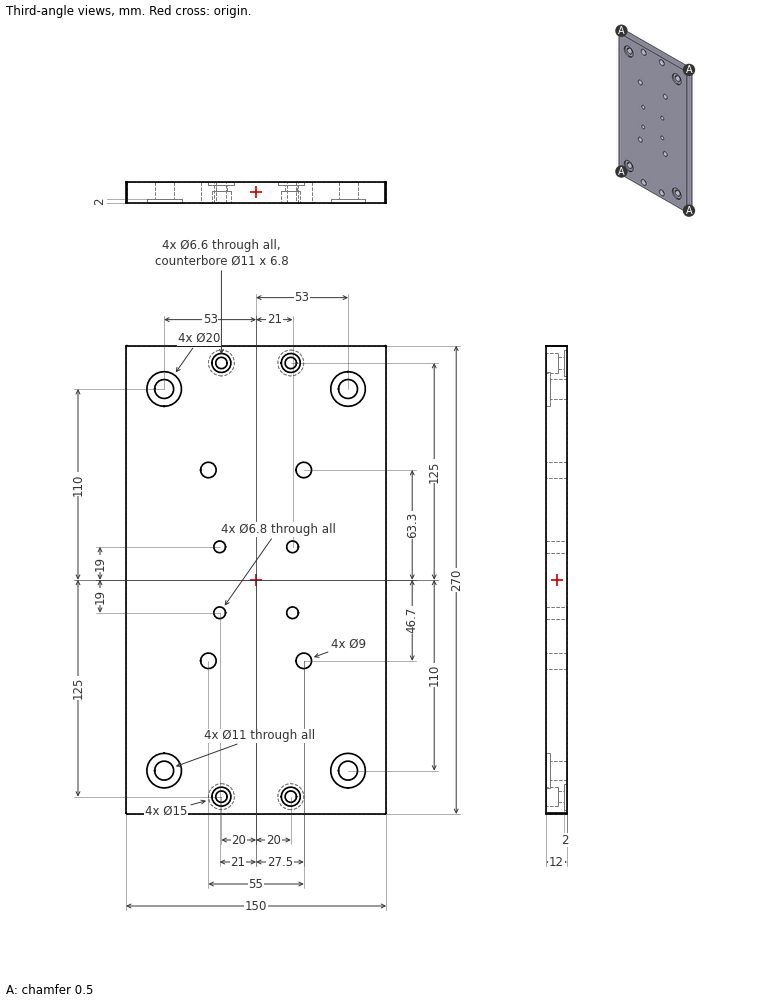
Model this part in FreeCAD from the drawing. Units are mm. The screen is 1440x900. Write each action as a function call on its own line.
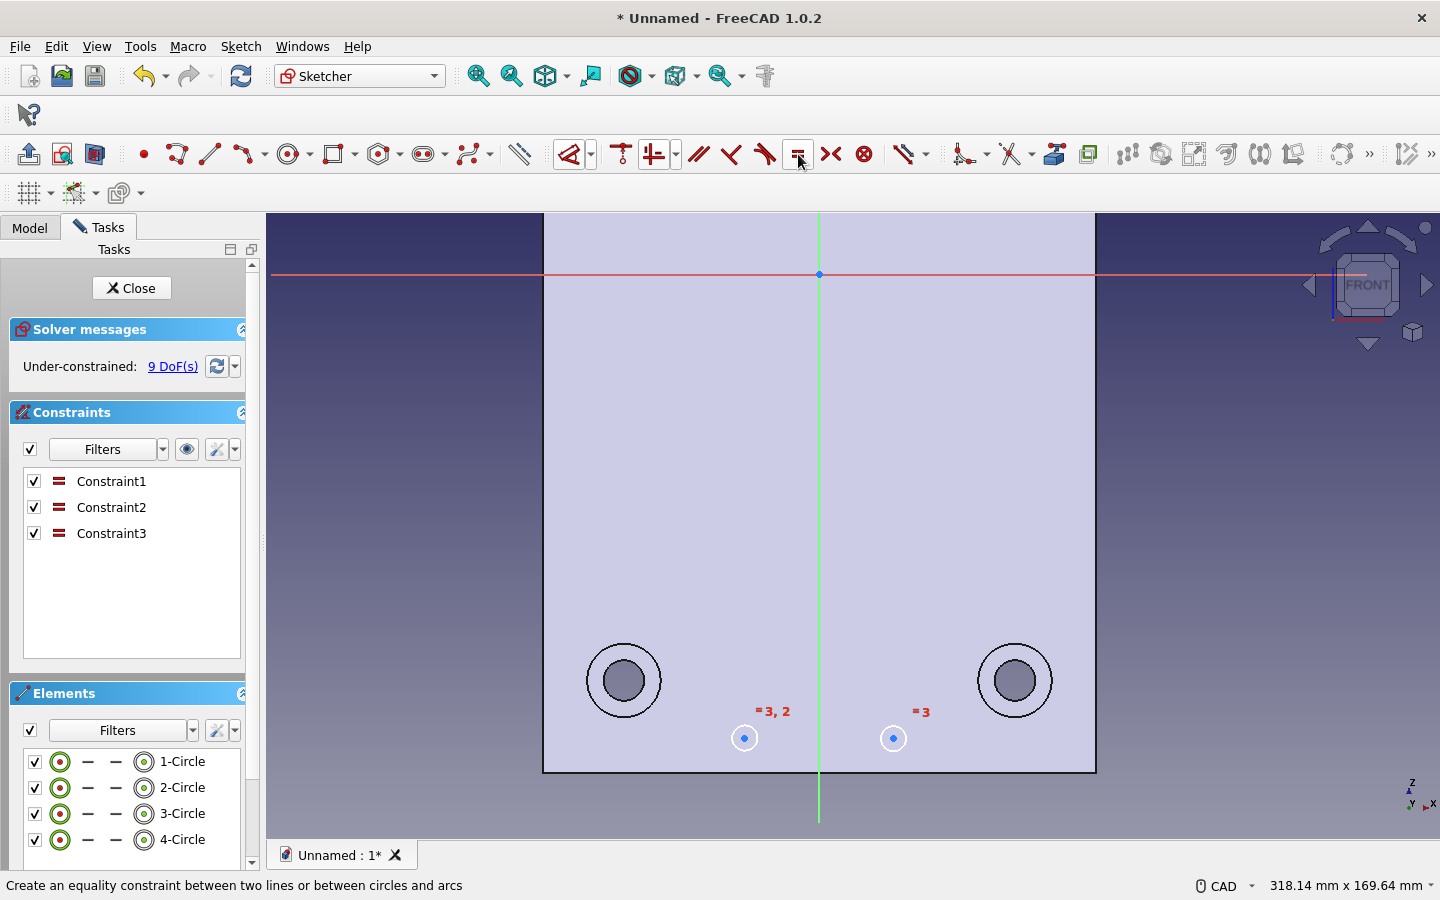
scroll(756, 731, down, 4)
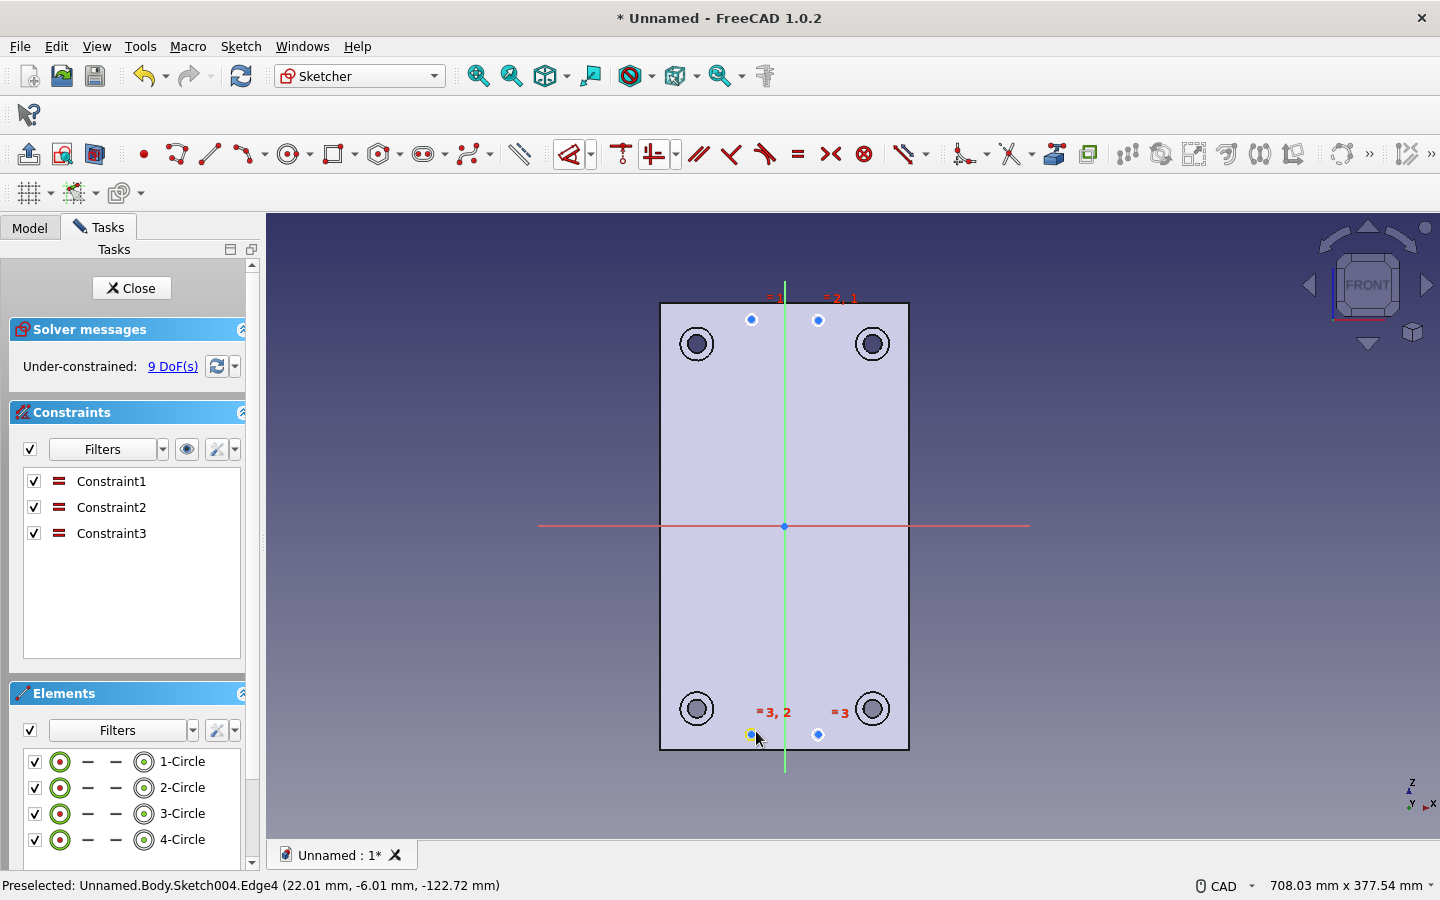
click(752, 320)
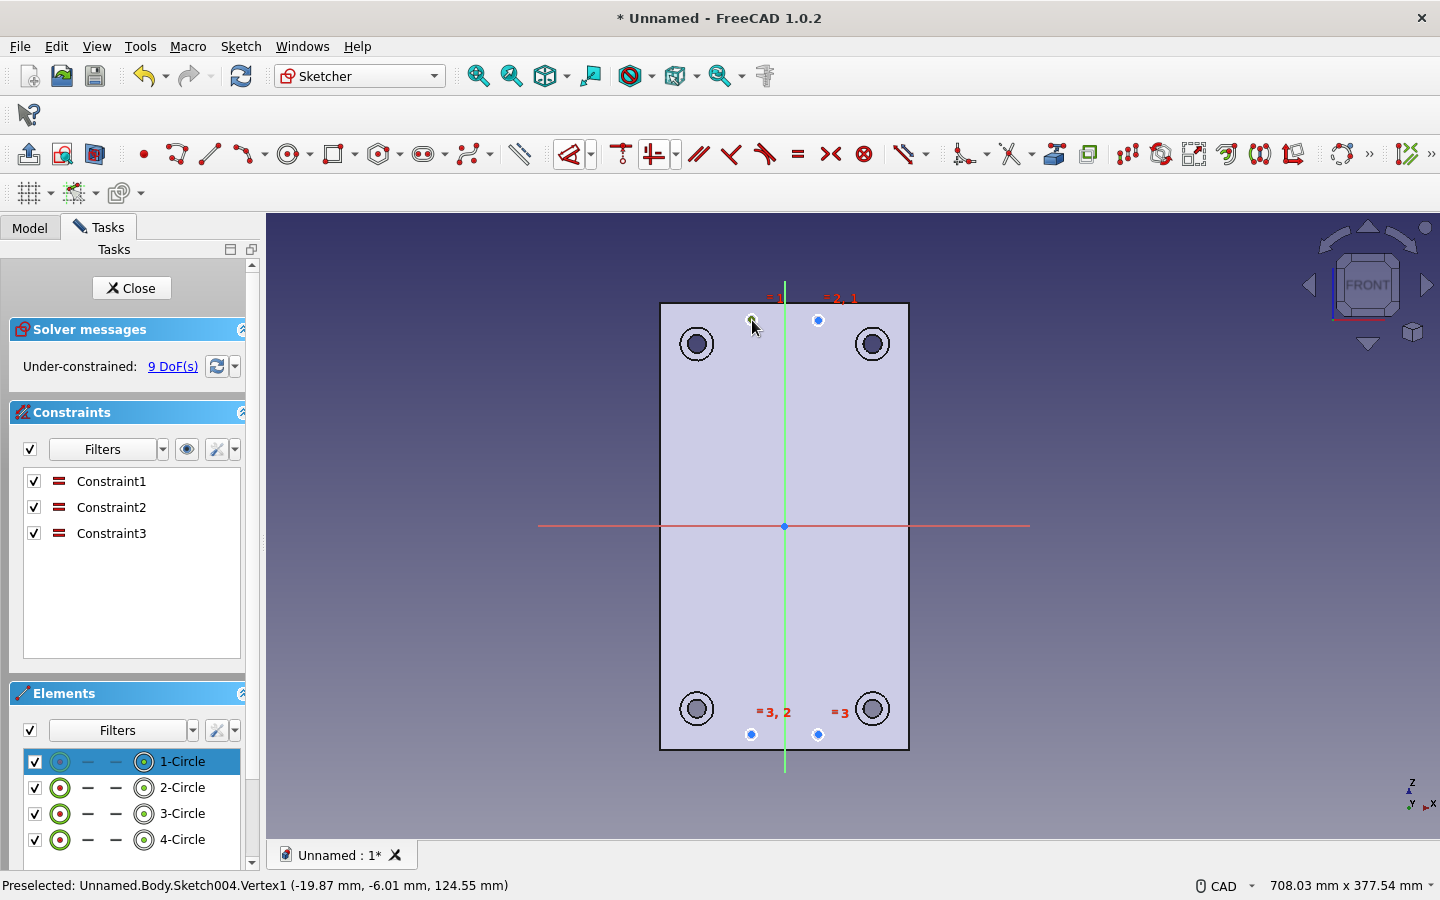
click(818, 320)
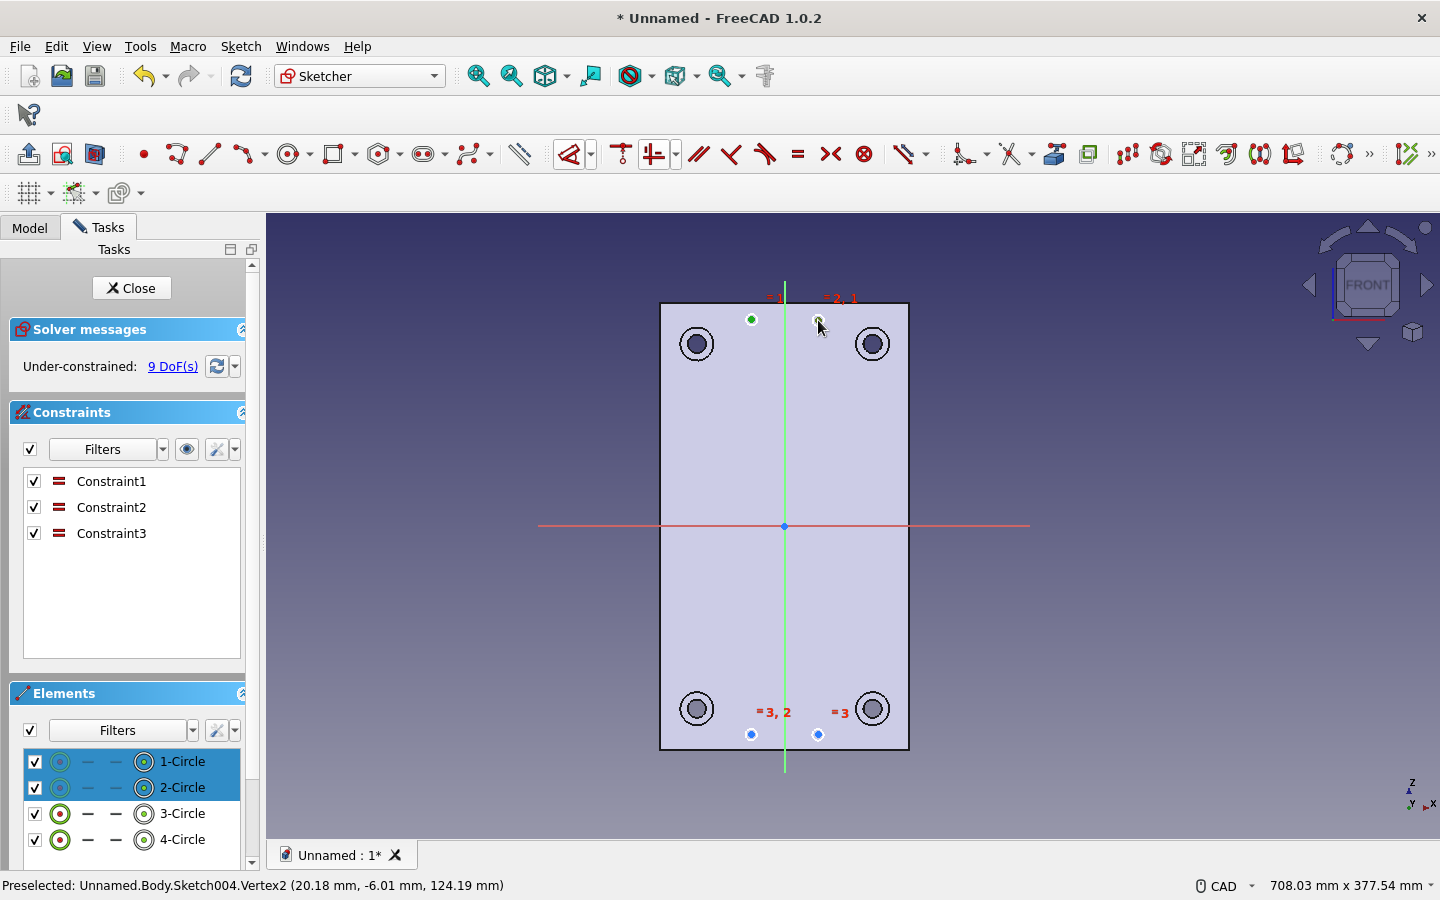
key(h)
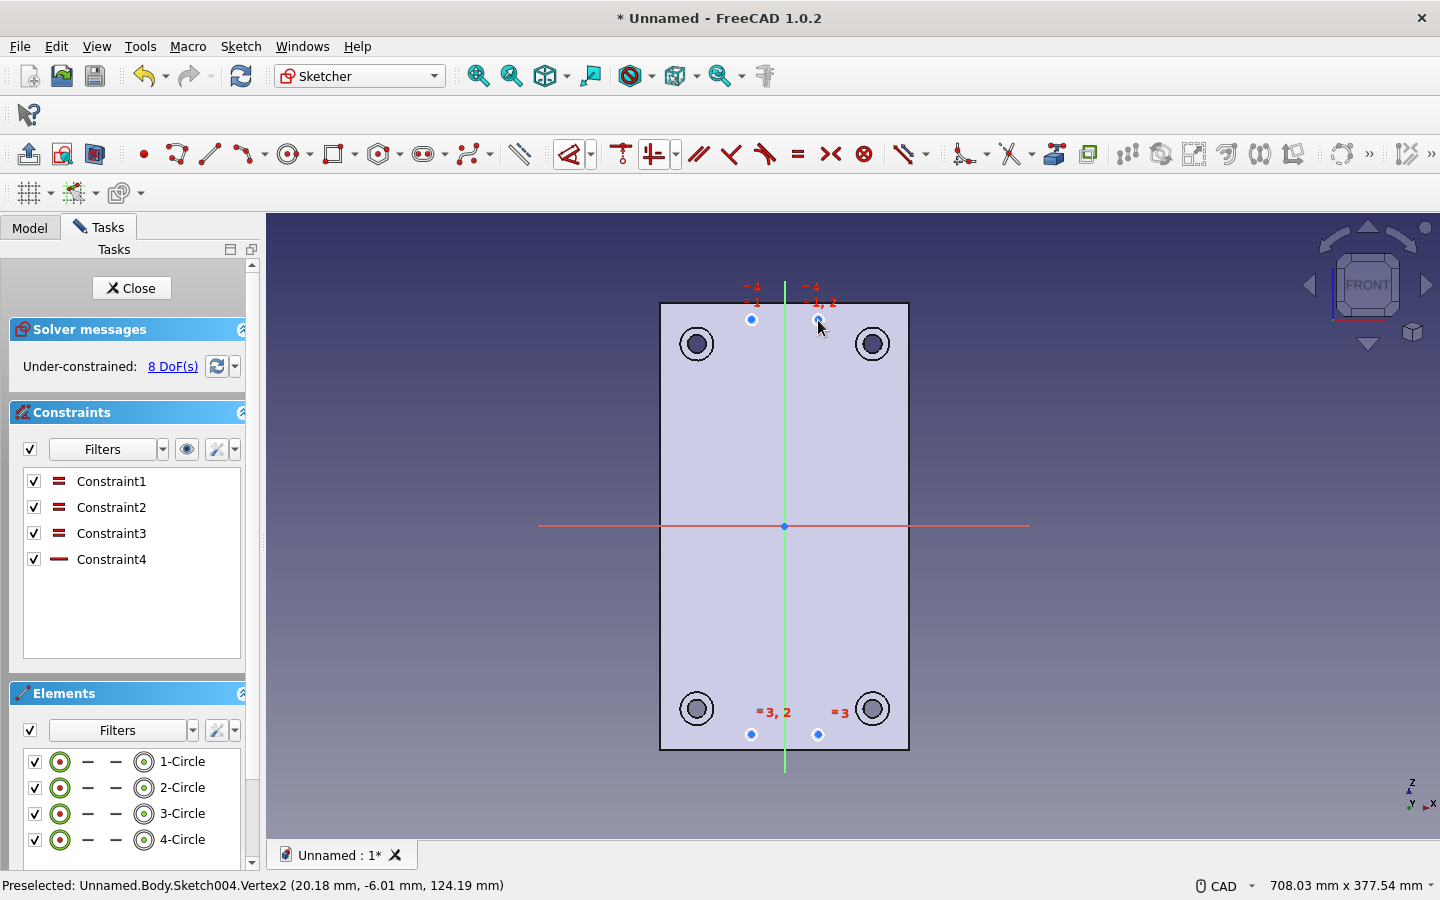
click(752, 320)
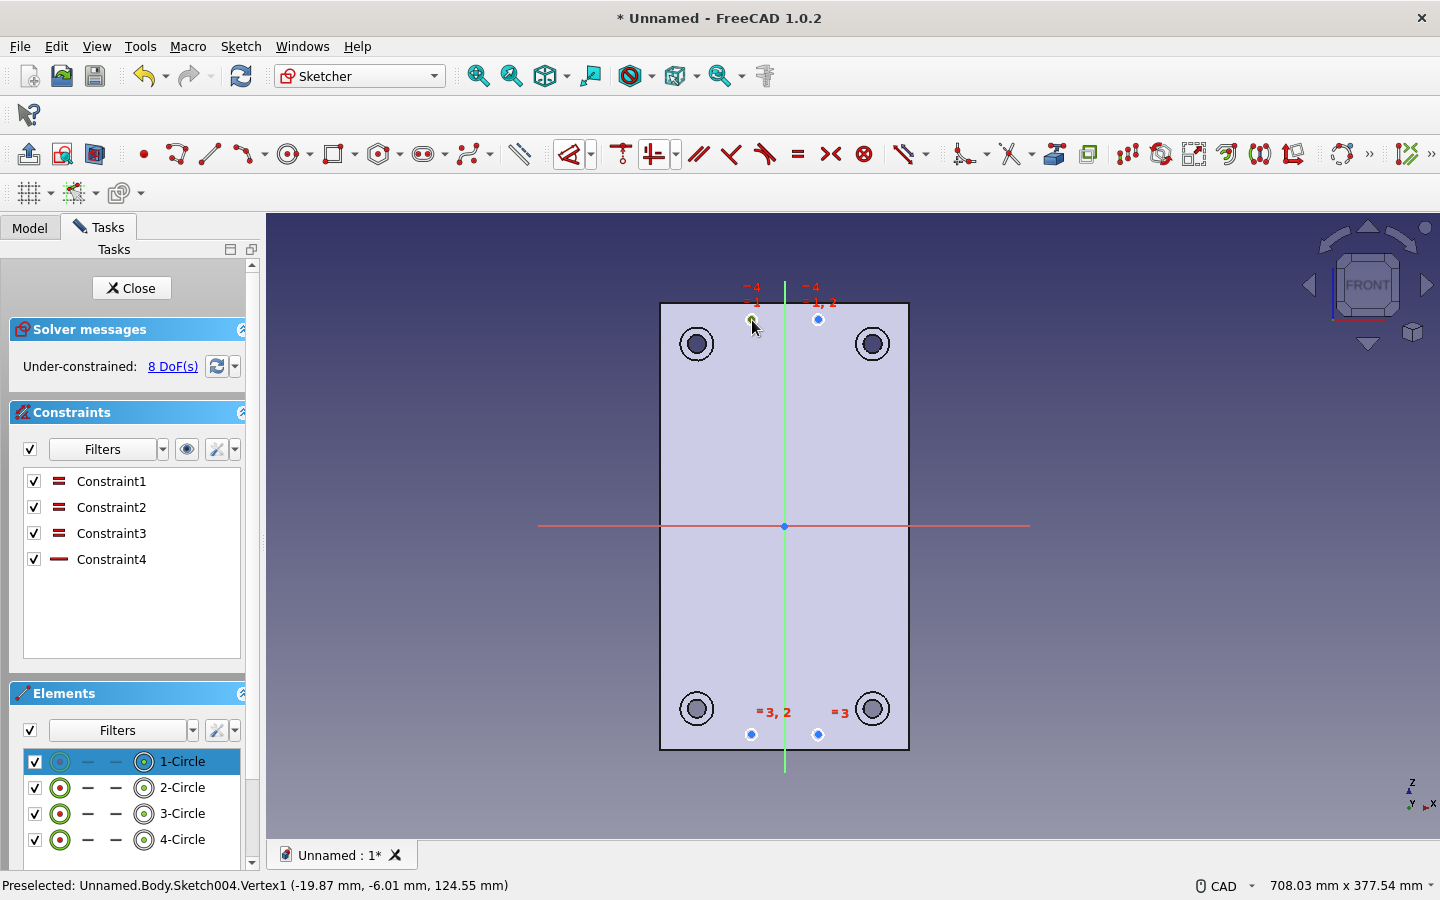
click(751, 735)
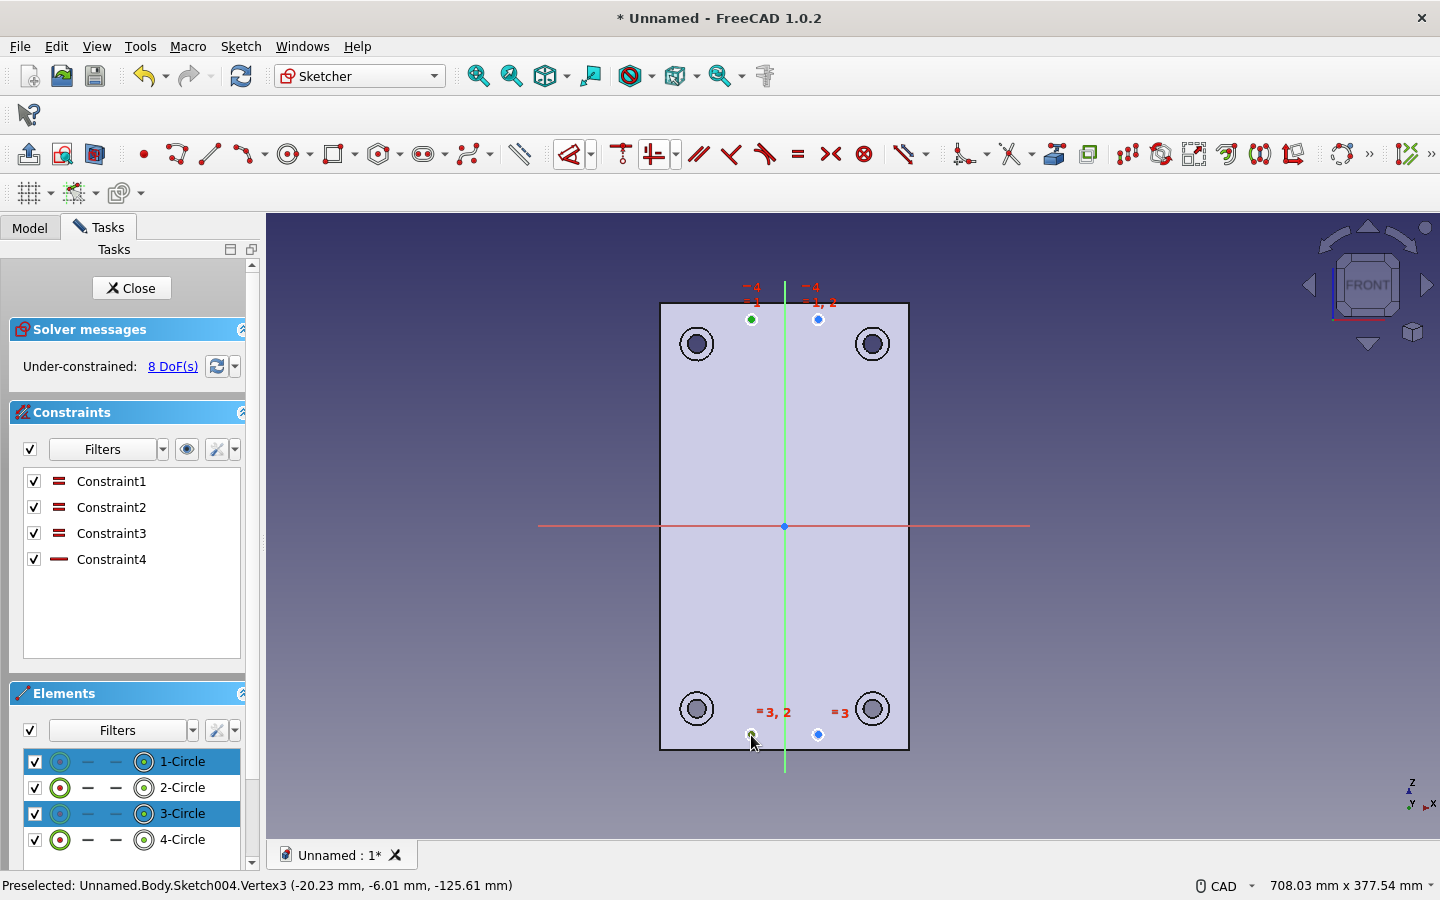
key(v)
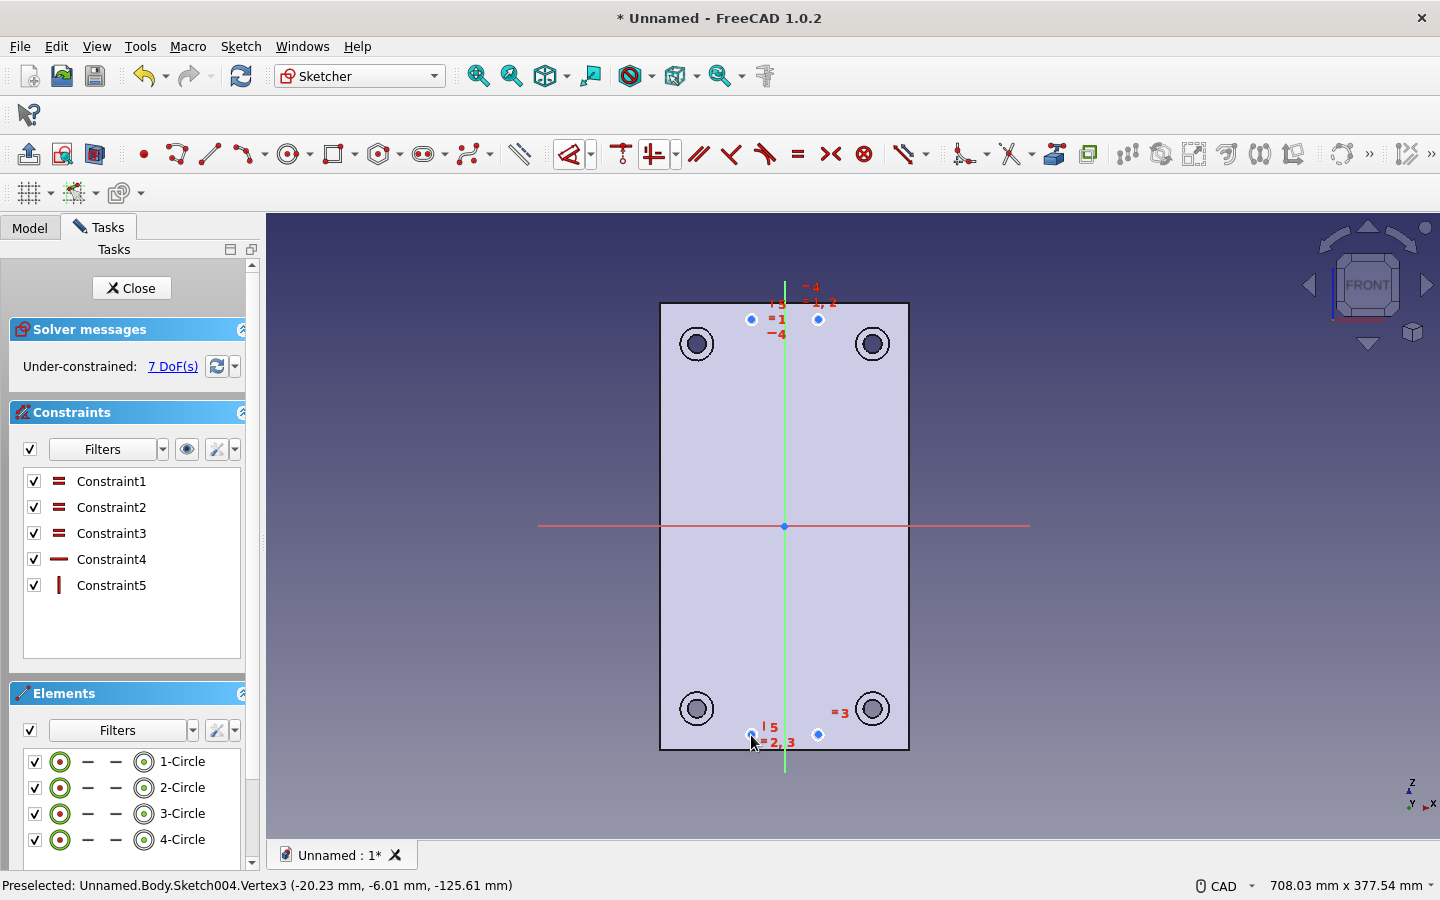
click(818, 320)